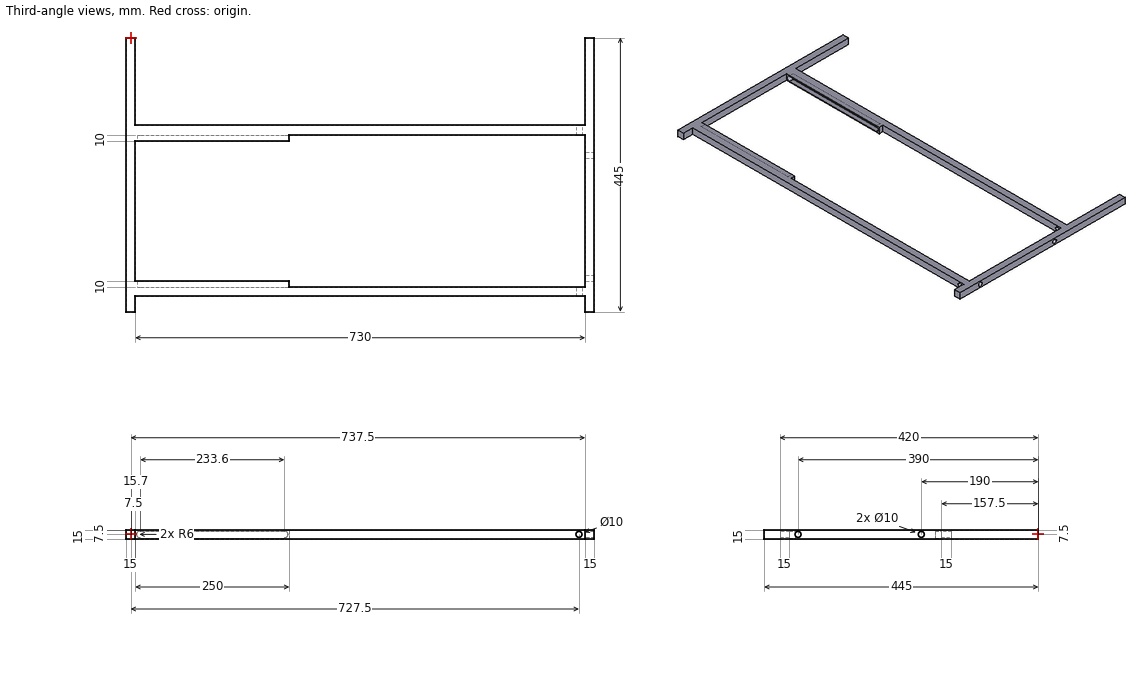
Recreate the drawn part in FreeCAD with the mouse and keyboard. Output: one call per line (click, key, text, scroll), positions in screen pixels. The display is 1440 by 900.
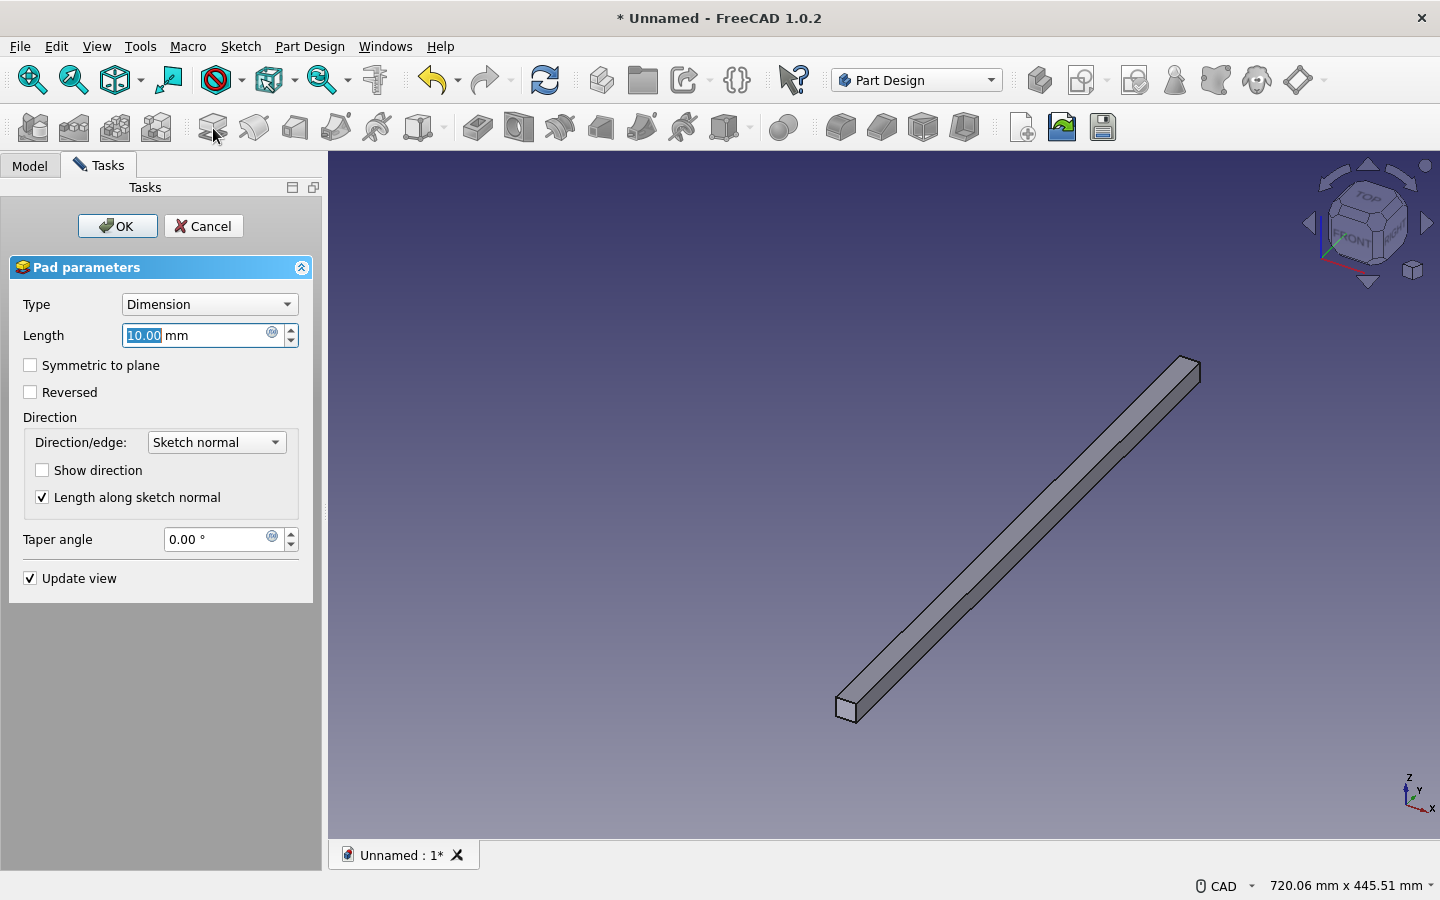
text(445)
key(Tab)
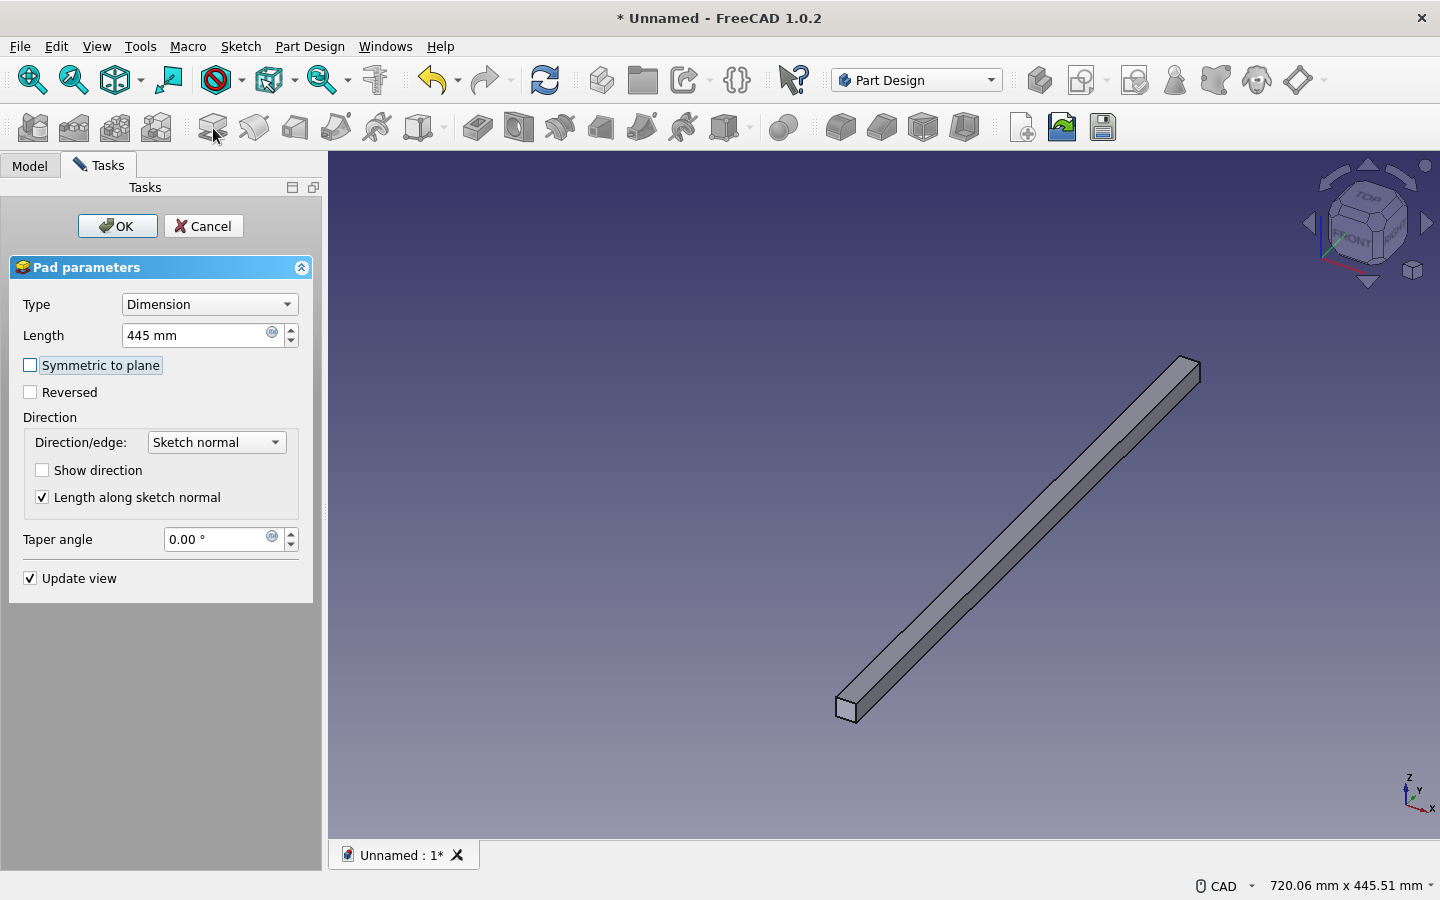
click(118, 226)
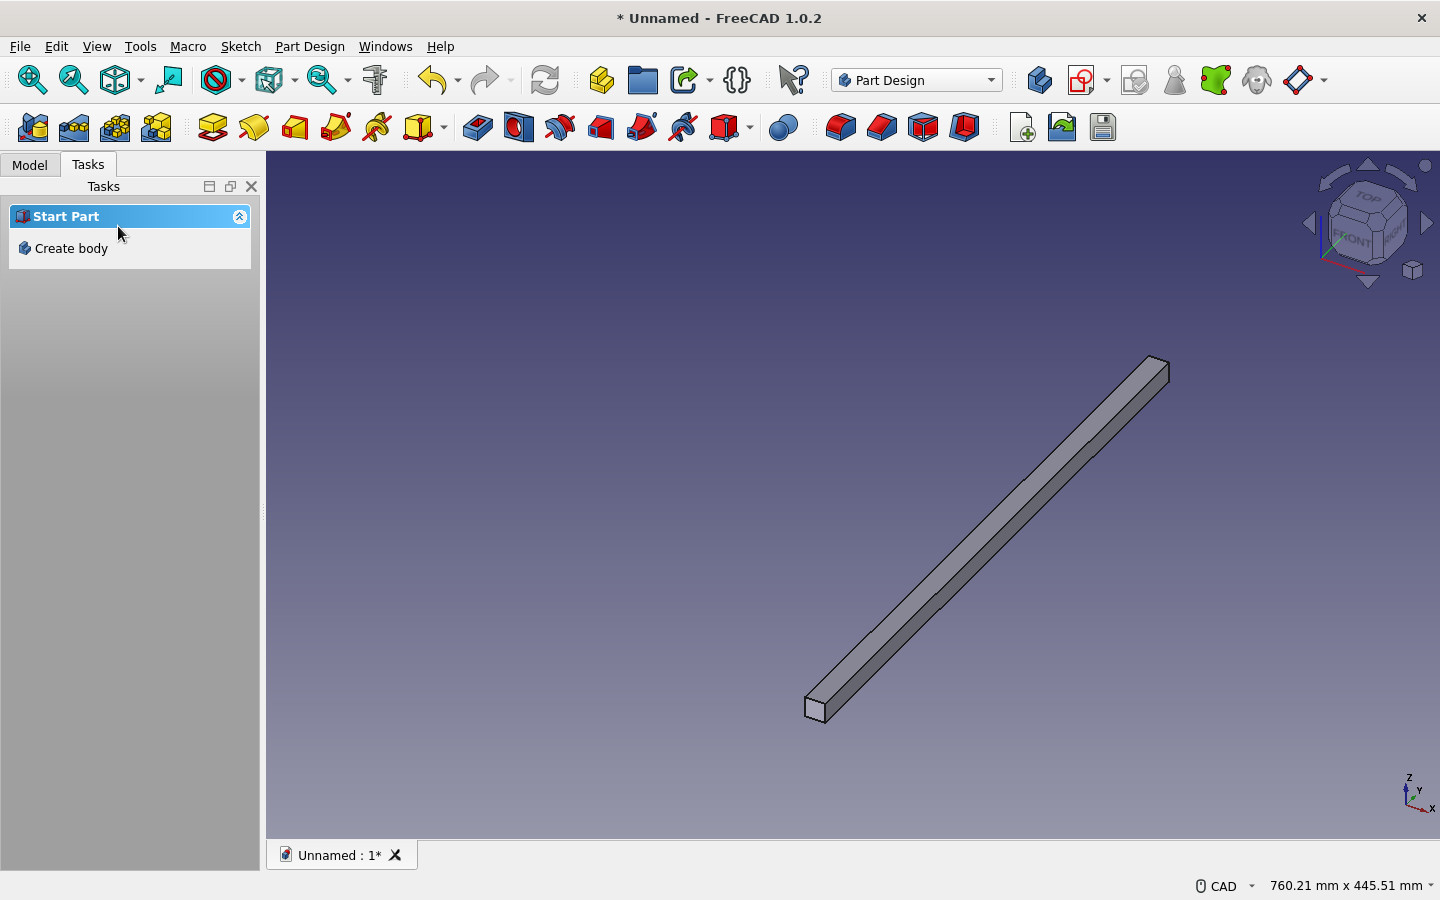
click(33, 80)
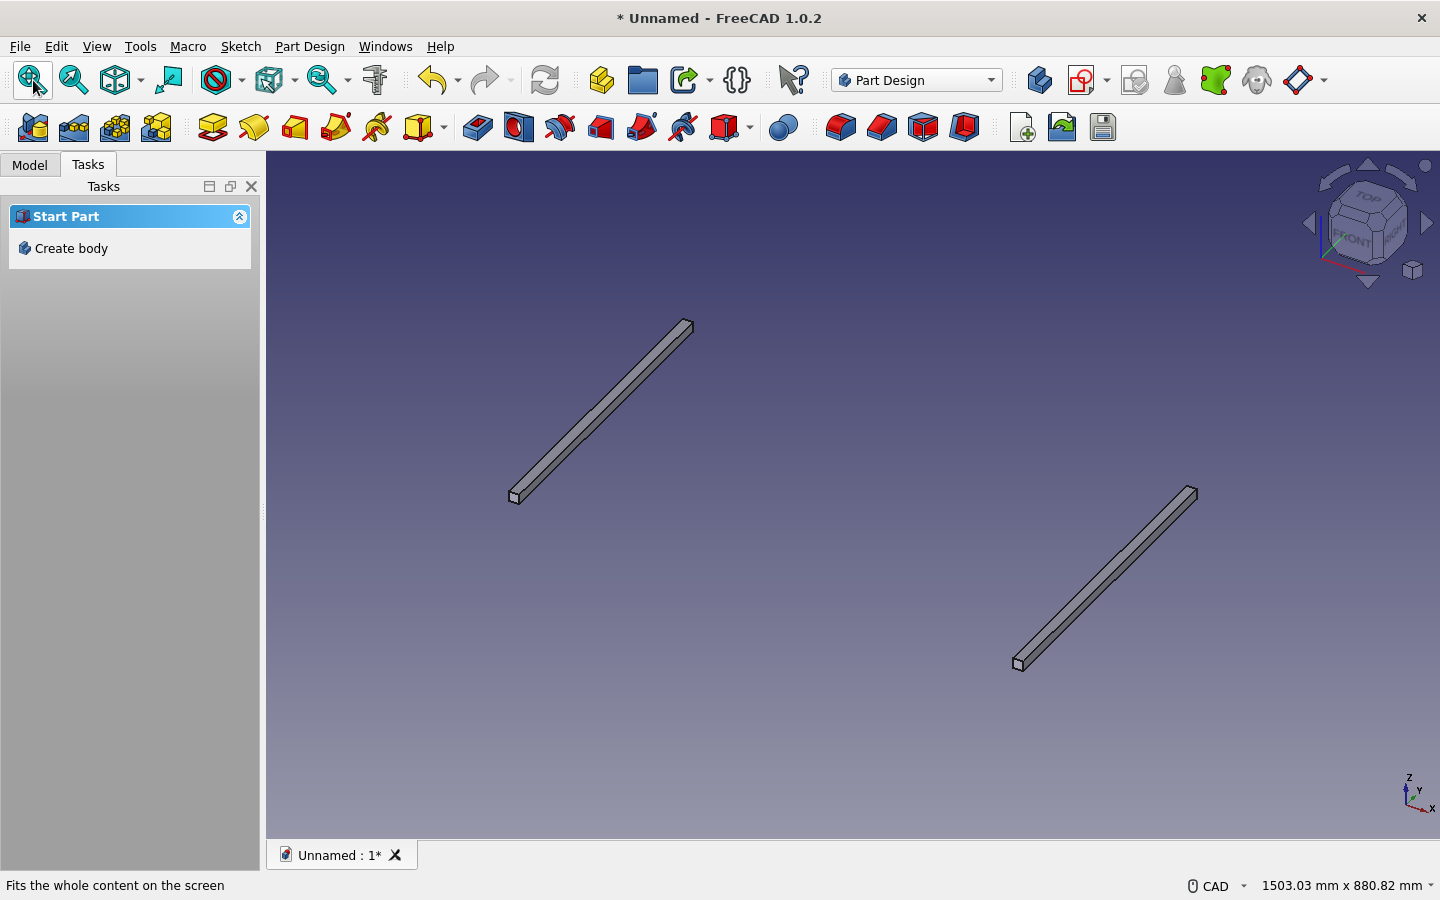
click(30, 164)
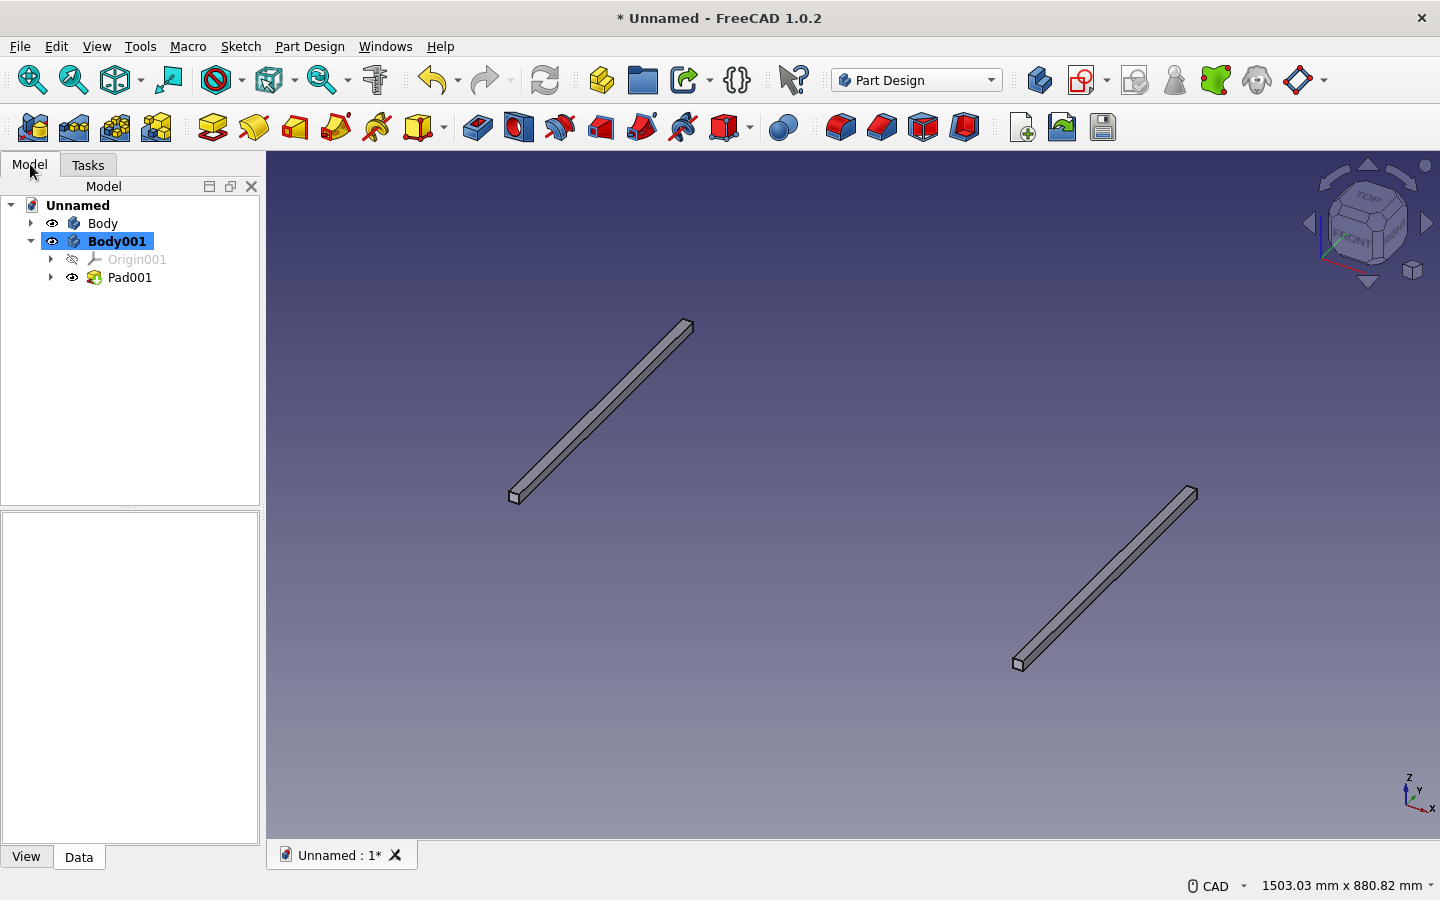
double_click(97, 223)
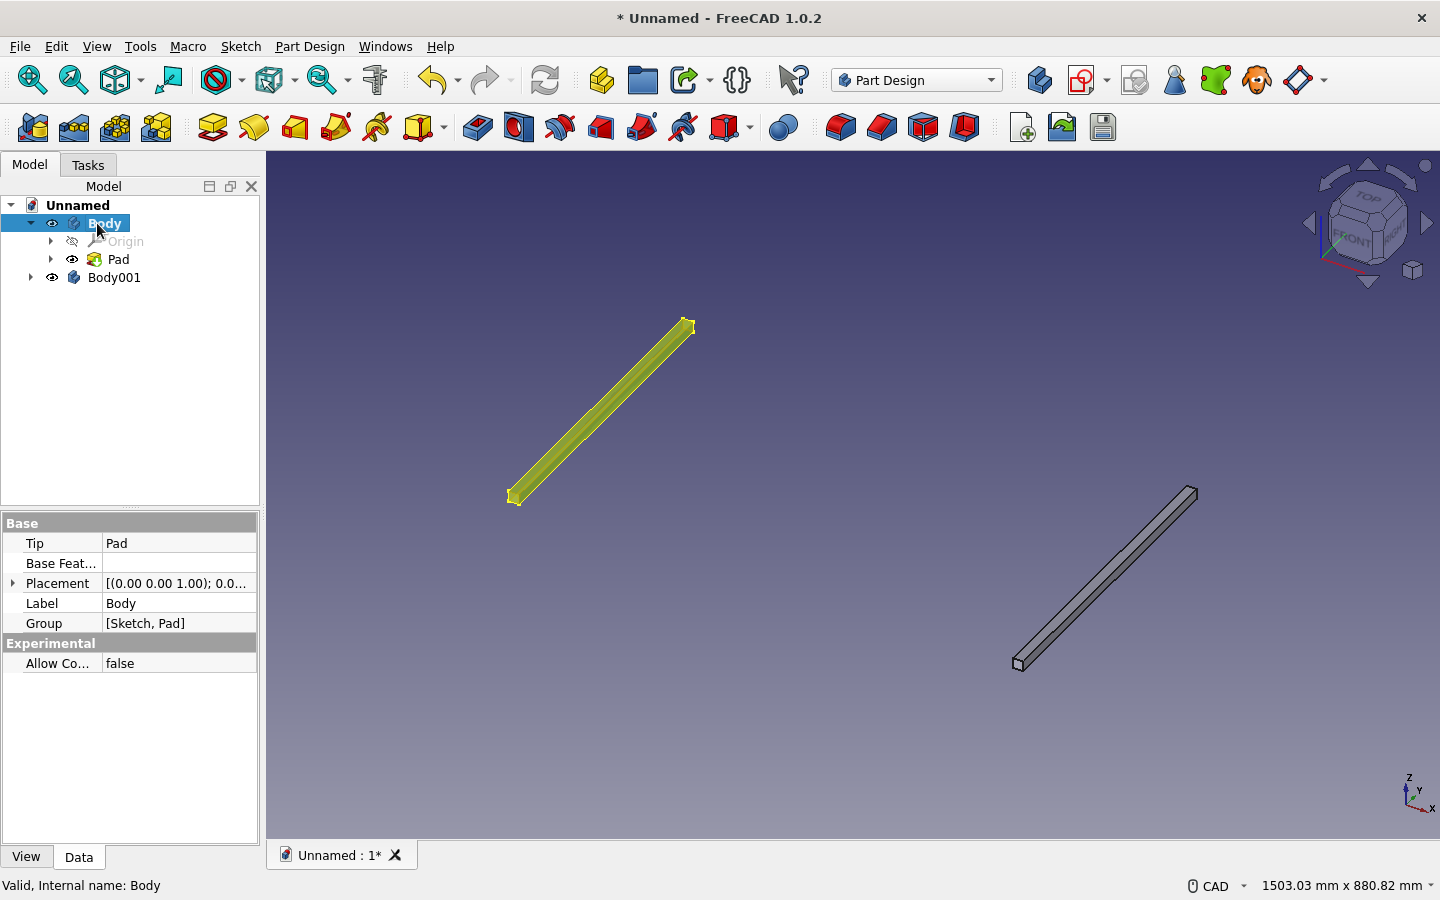
click(97, 223)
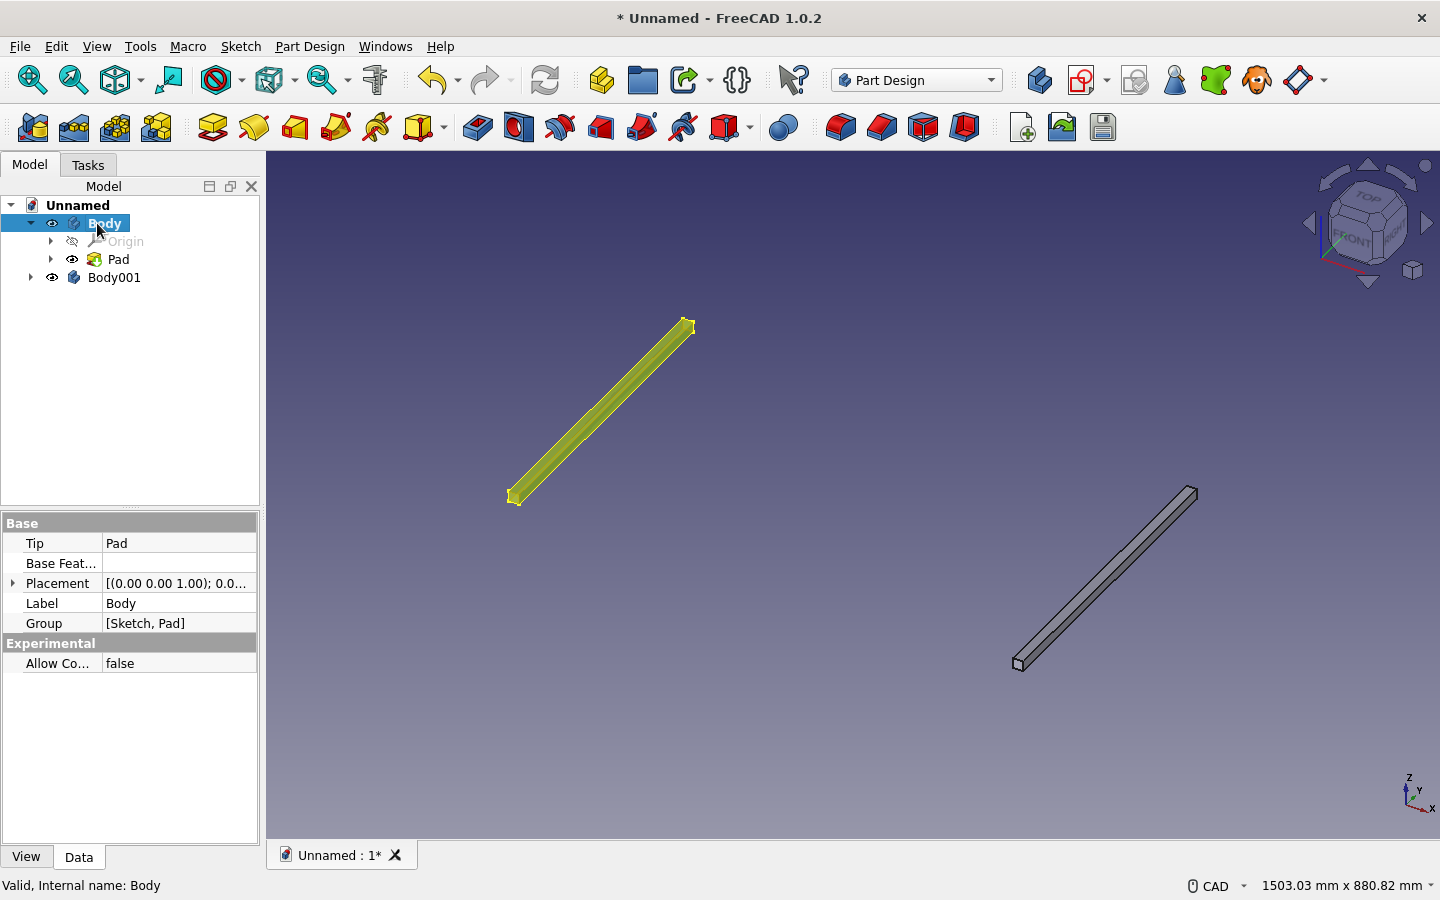
click(148, 663)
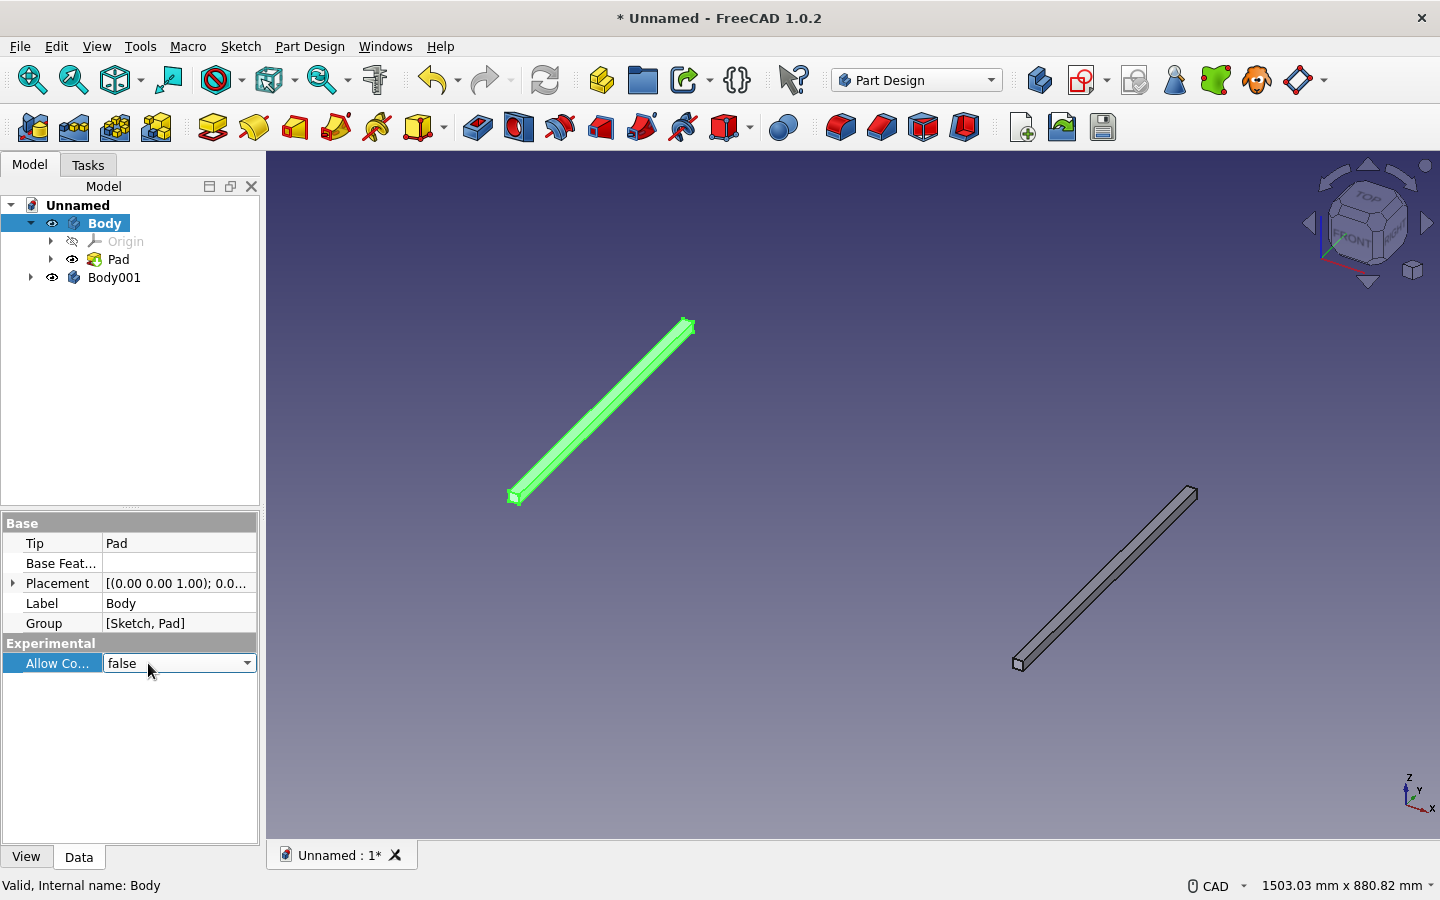
click(148, 663)